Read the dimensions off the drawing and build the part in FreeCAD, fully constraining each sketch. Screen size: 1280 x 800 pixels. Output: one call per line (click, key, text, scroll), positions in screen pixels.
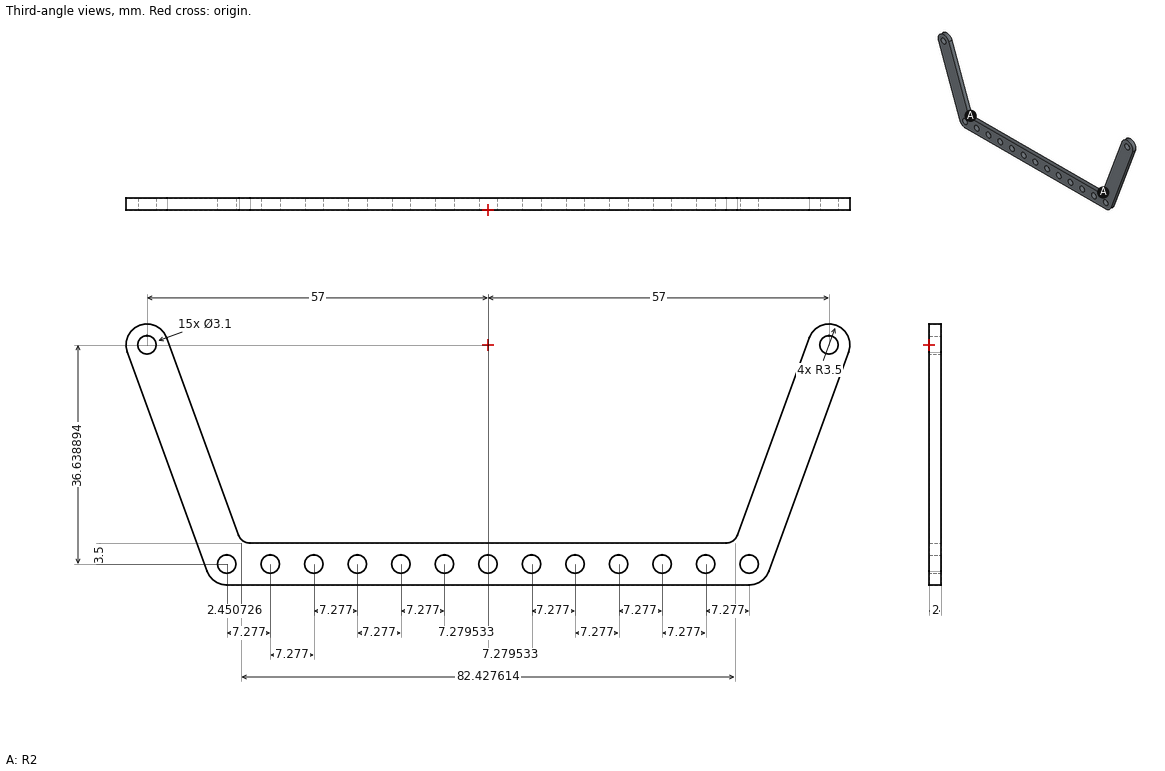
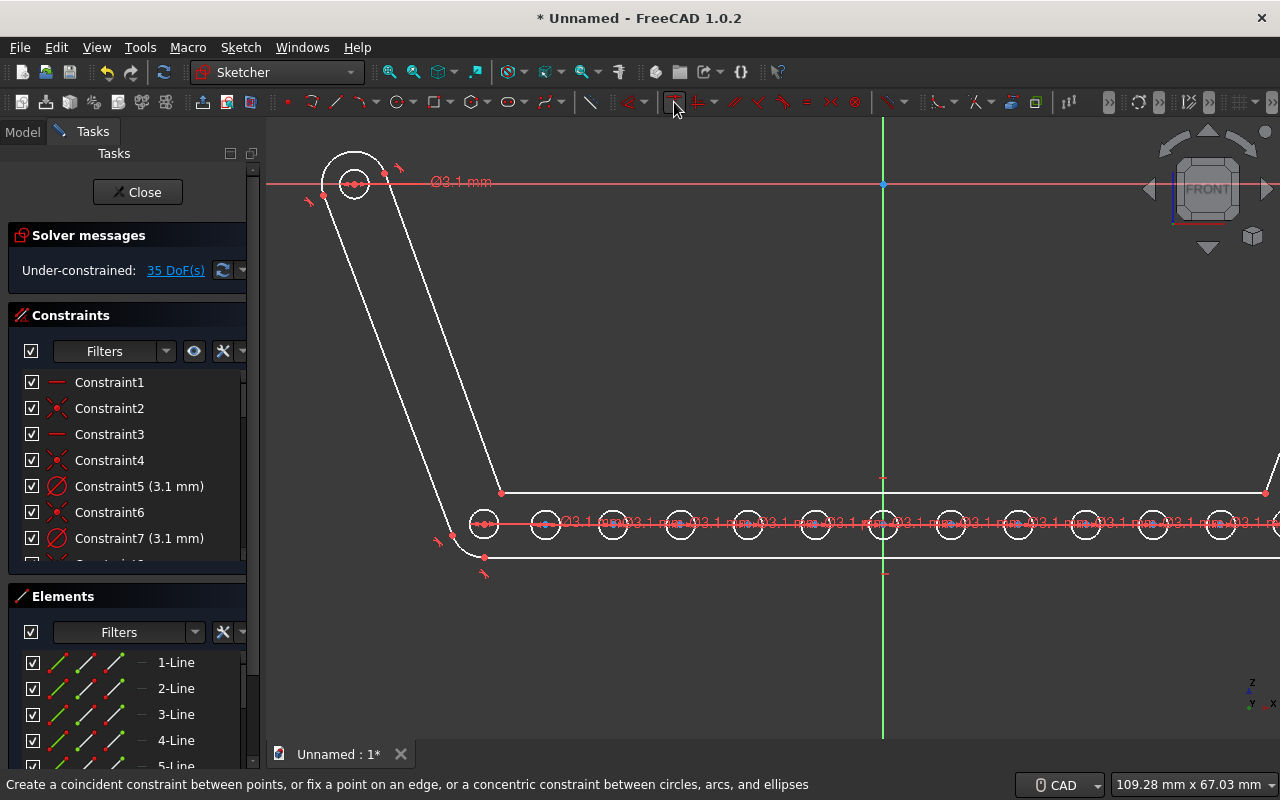
scroll(487, 517, down, 3)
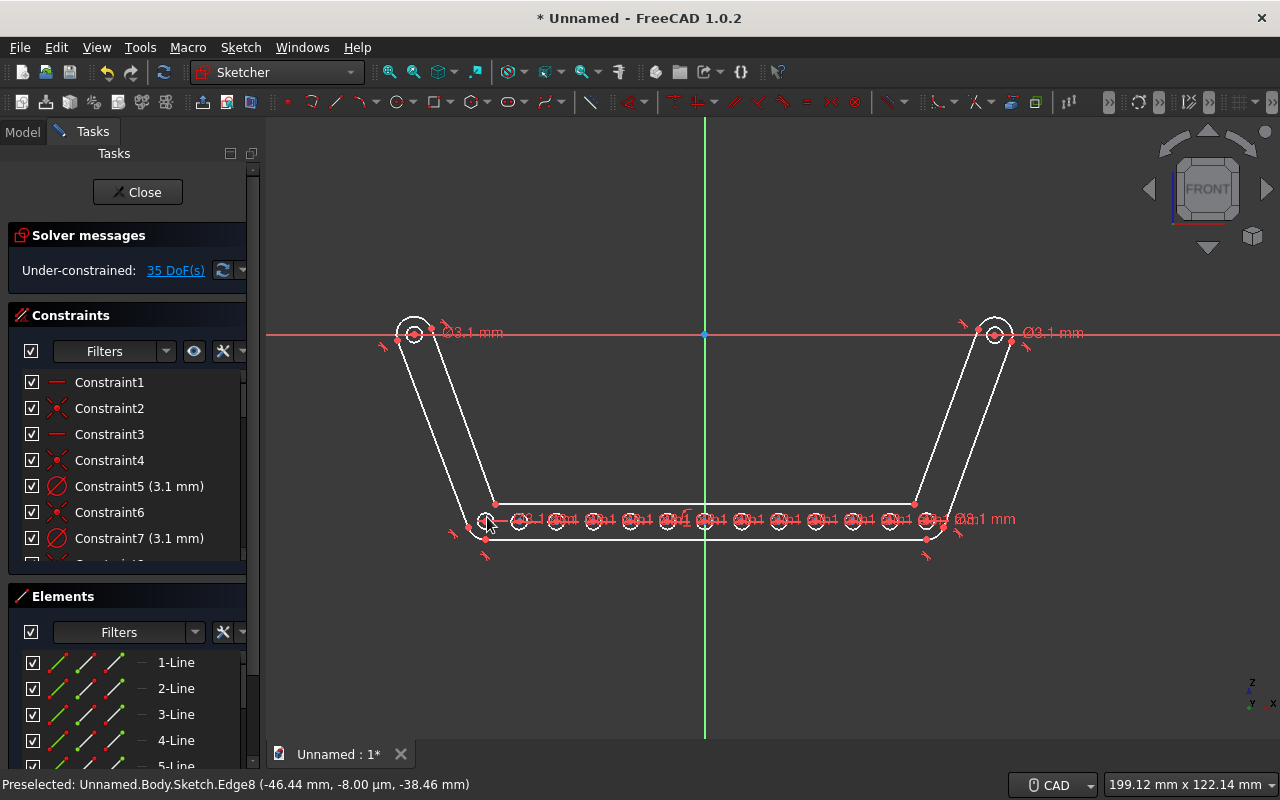
scroll(933, 538, up, 4)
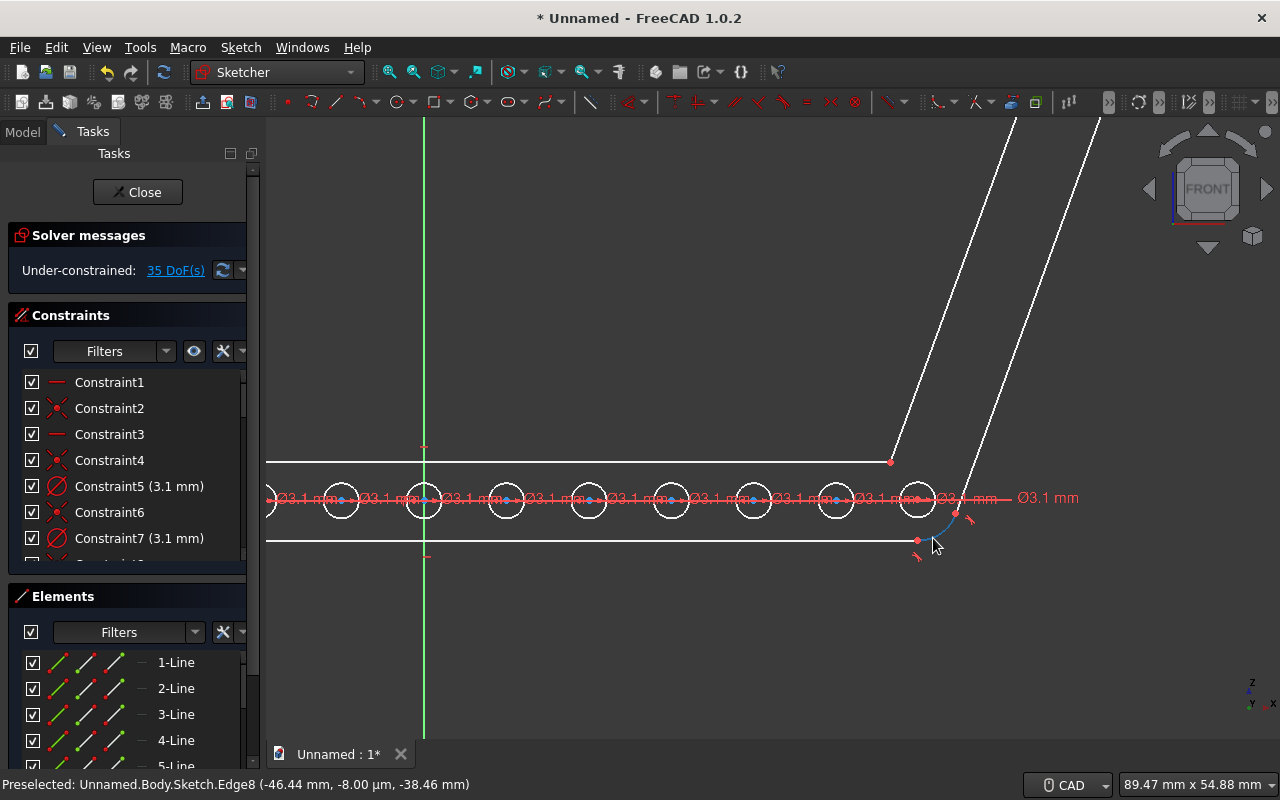
click(932, 538)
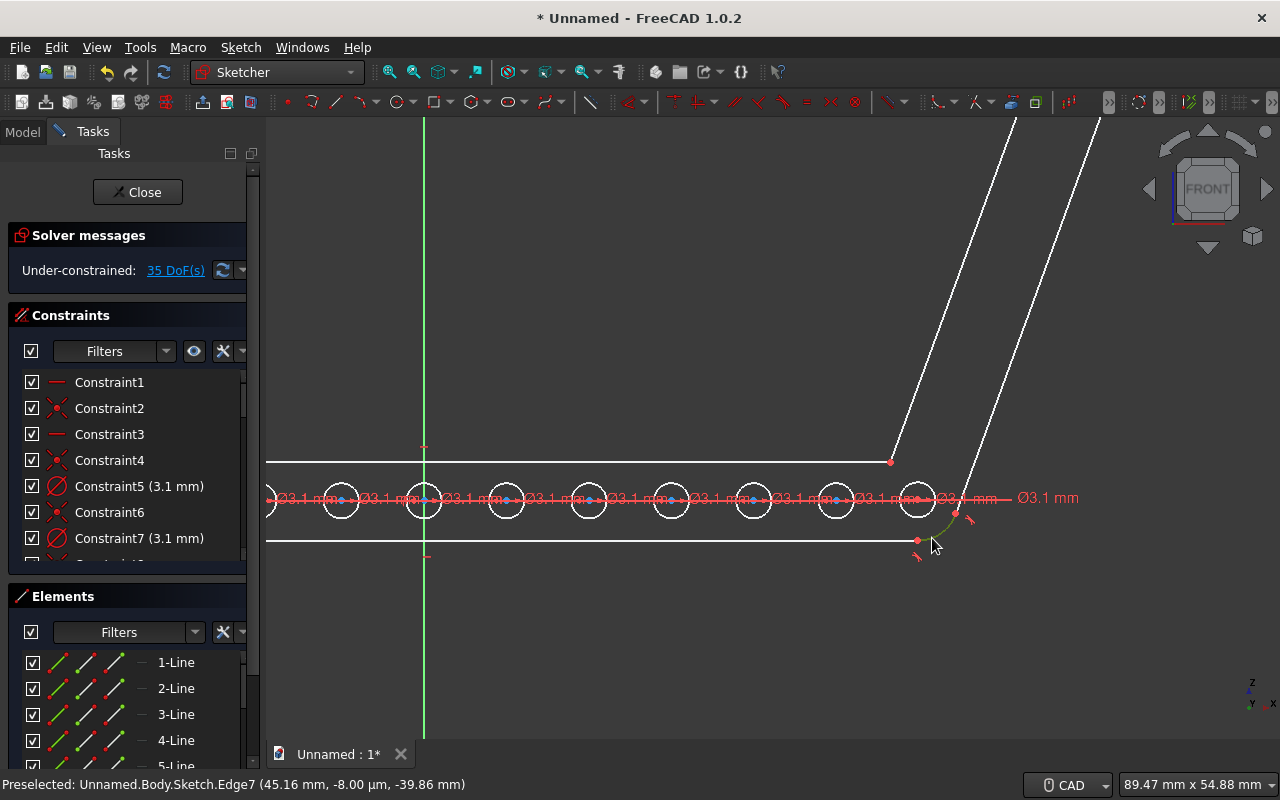
scroll(933, 538, down, 4)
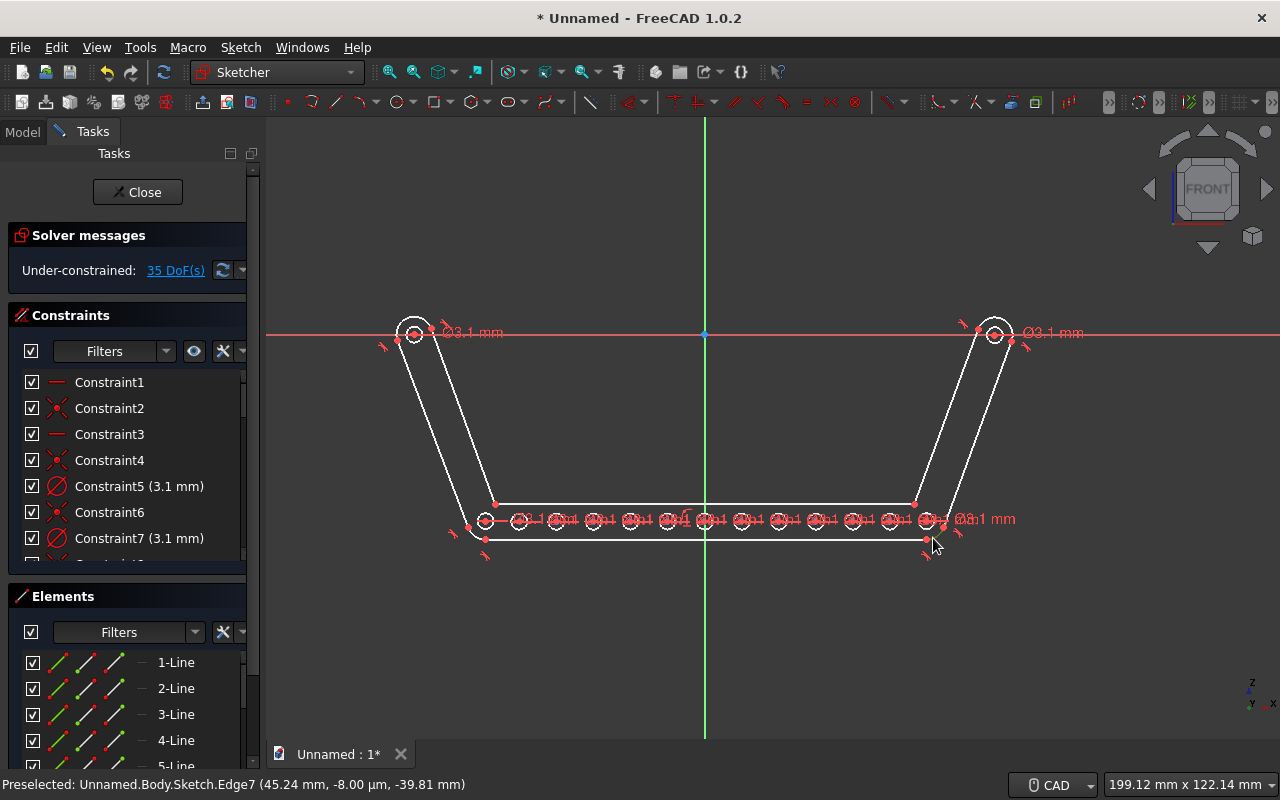
scroll(472, 533, up, 4)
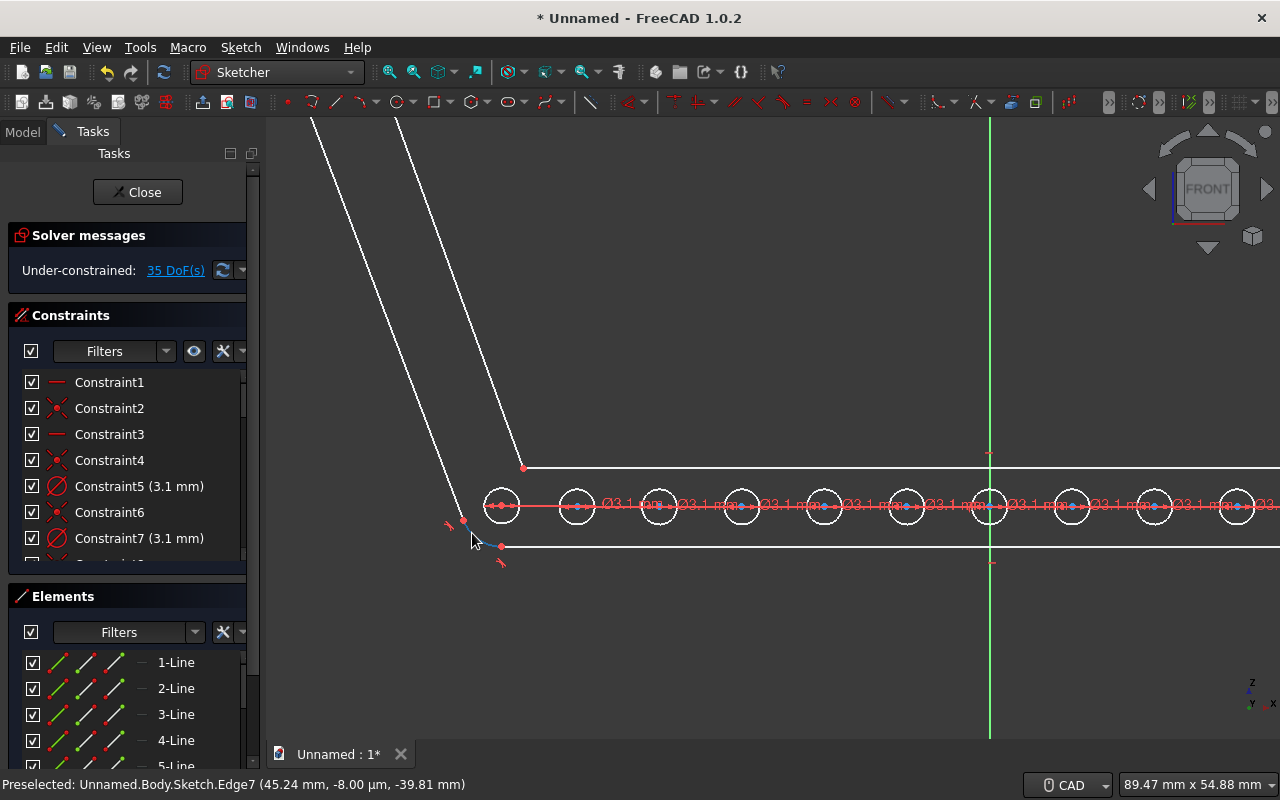
click(471, 533)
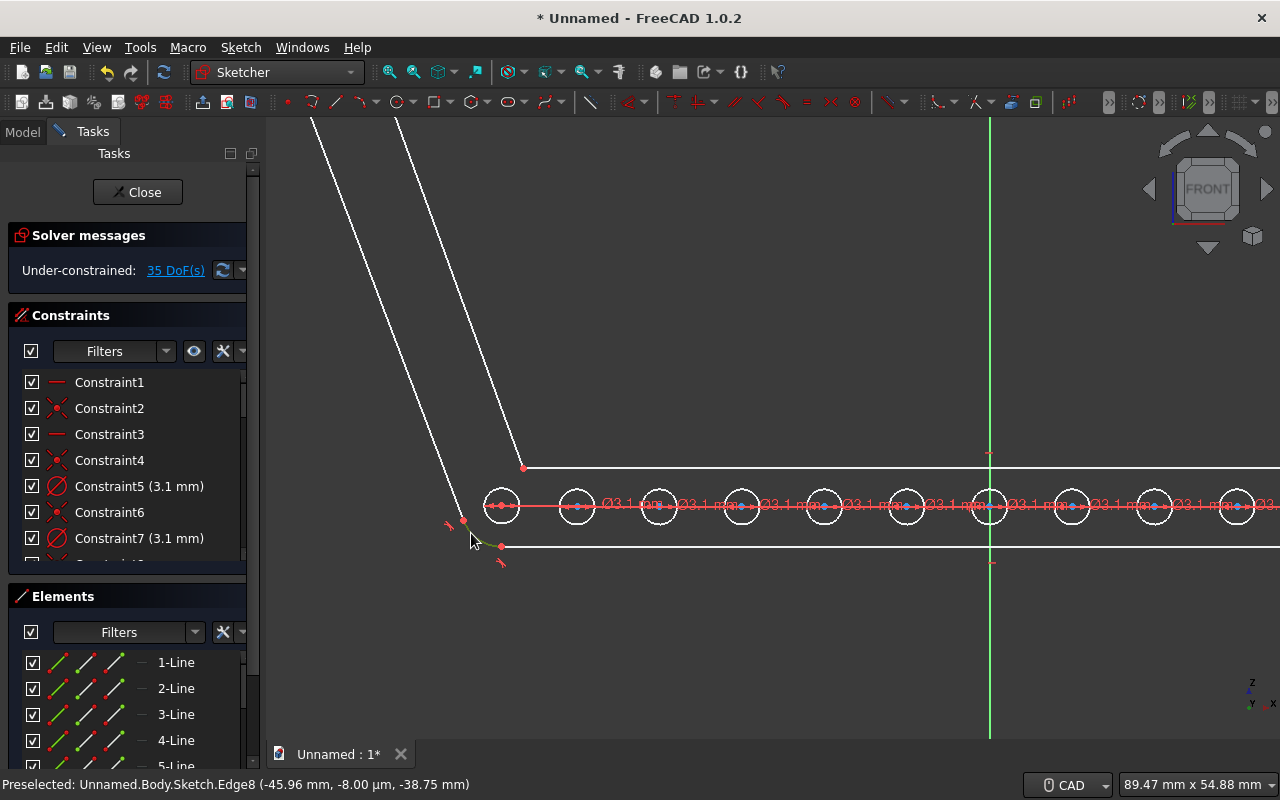
scroll(472, 533, down, 4)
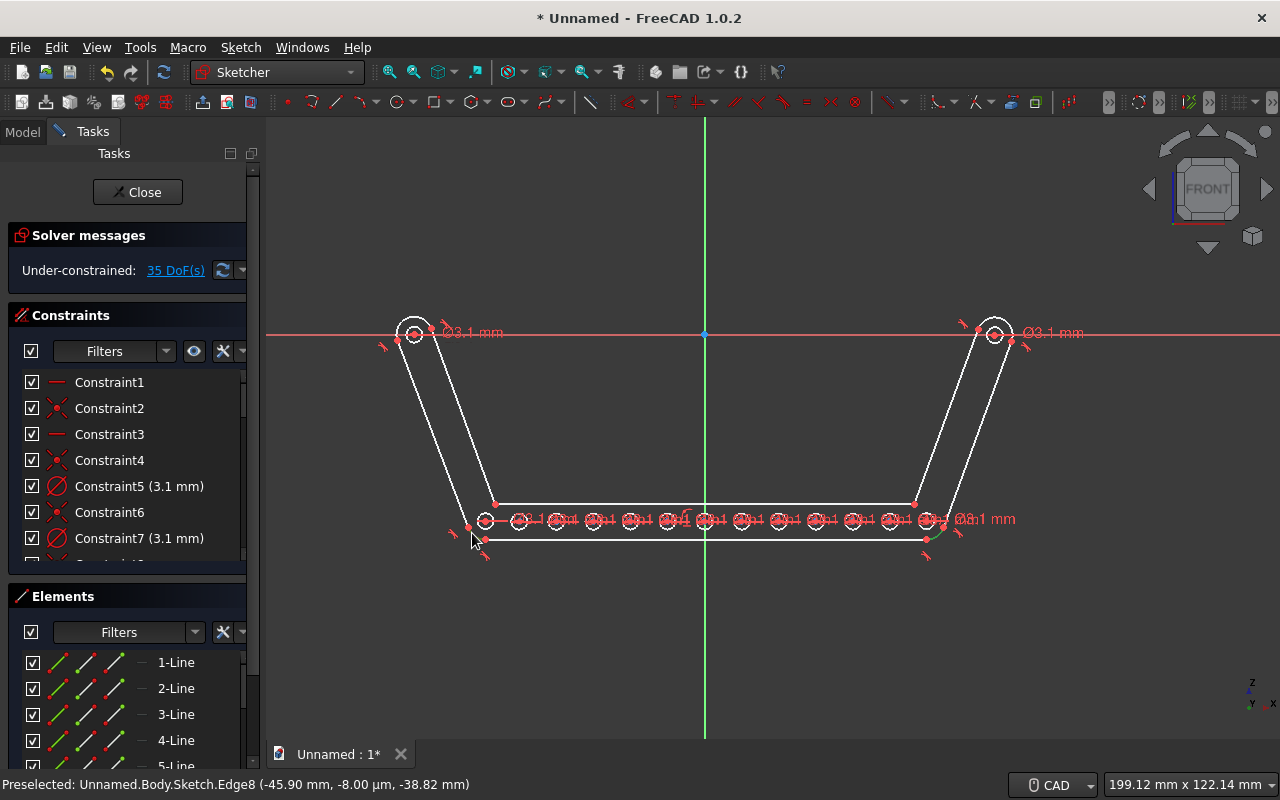
scroll(419, 317, up, 2)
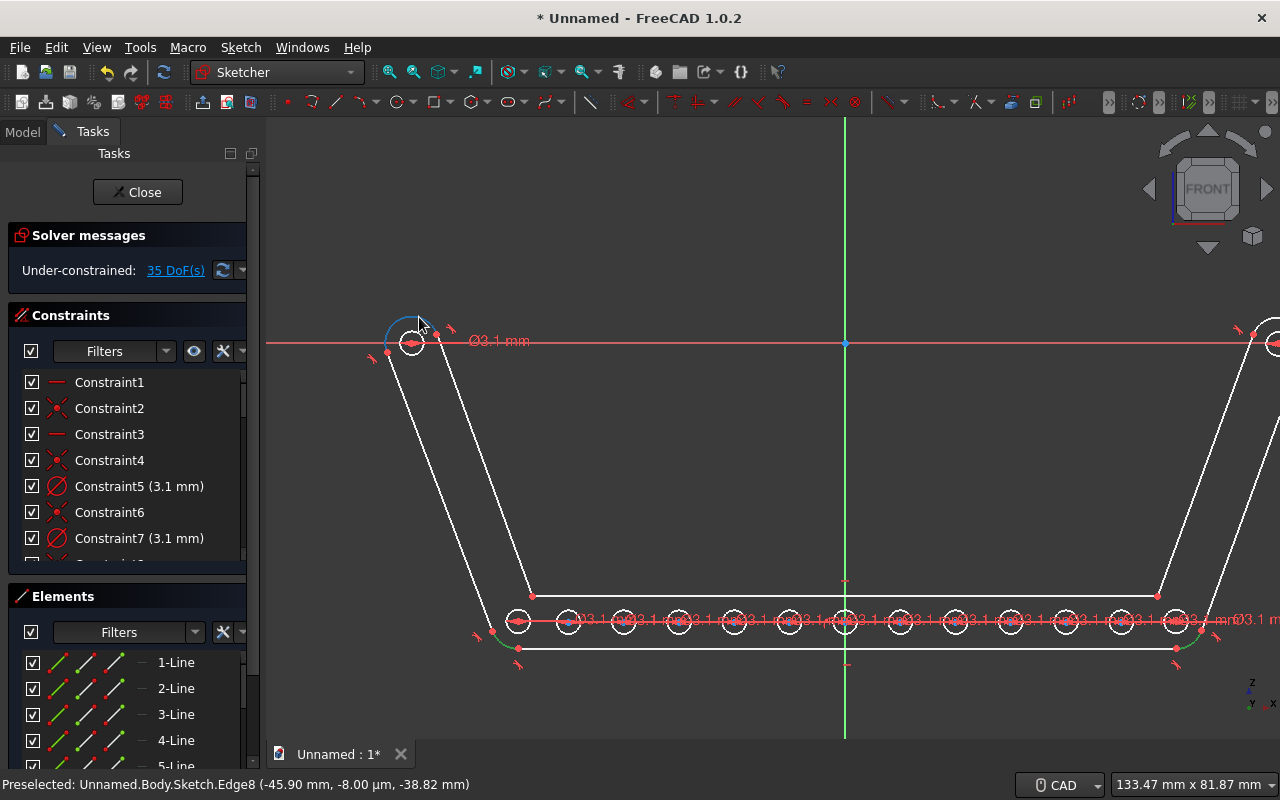
click(419, 318)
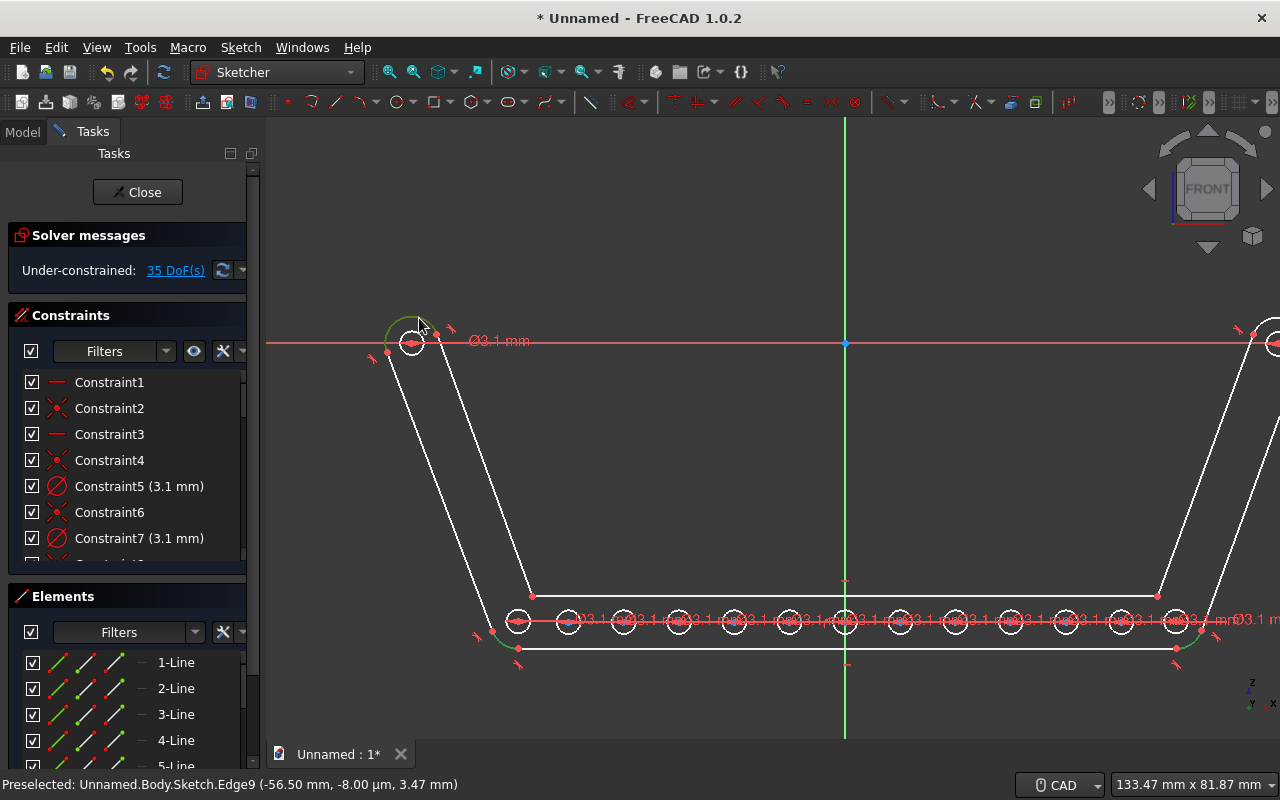
scroll(419, 316, down, 2)